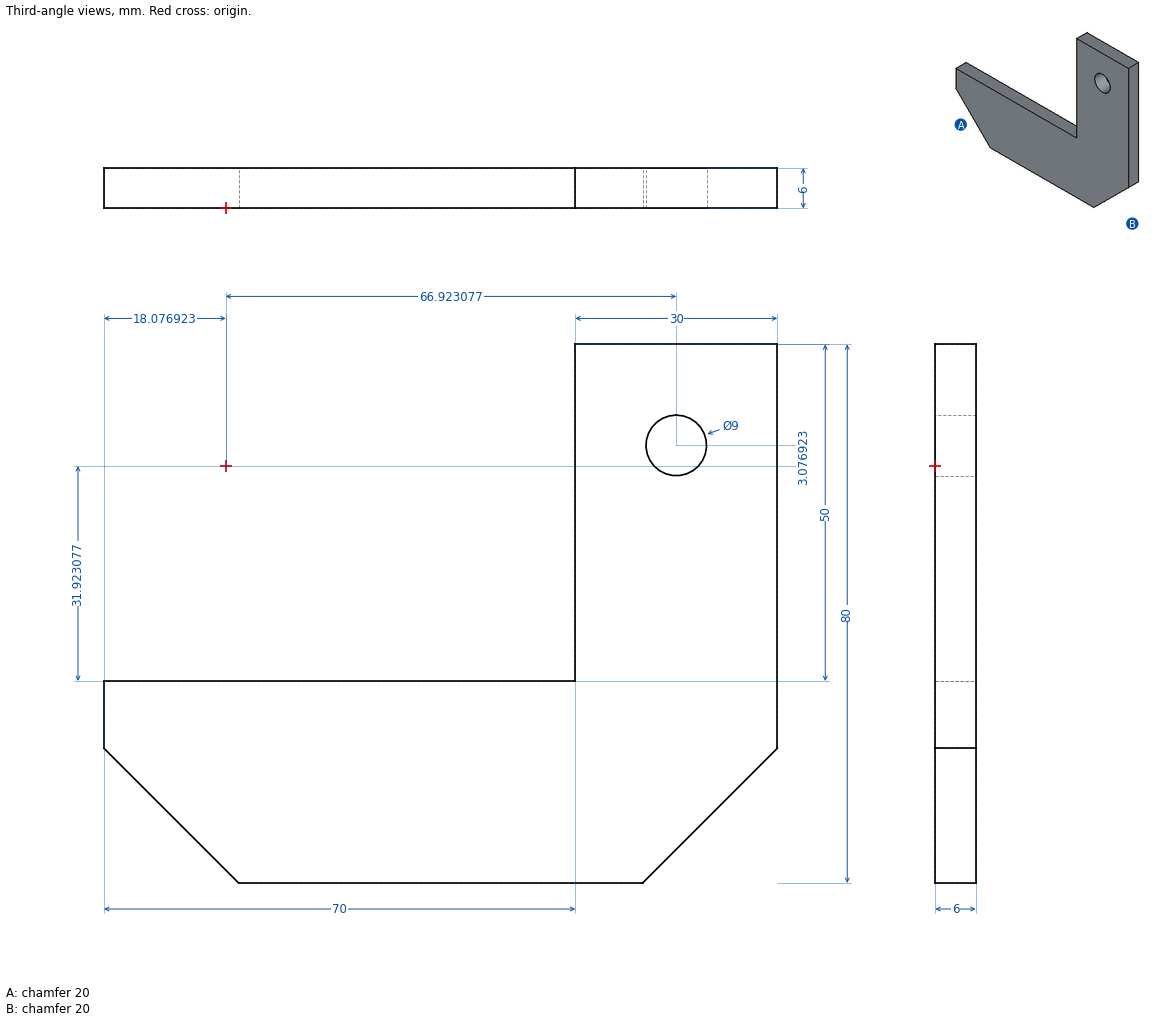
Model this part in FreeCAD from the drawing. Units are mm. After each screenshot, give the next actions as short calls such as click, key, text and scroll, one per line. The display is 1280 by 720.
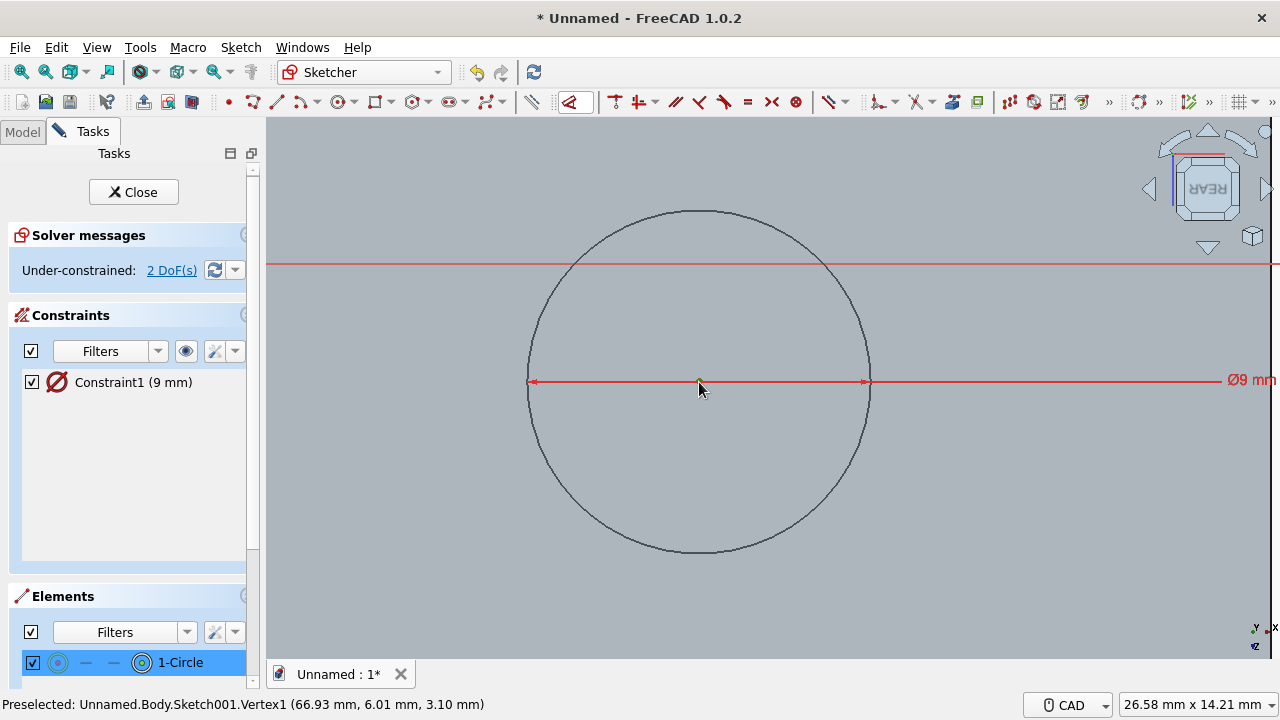
key(i)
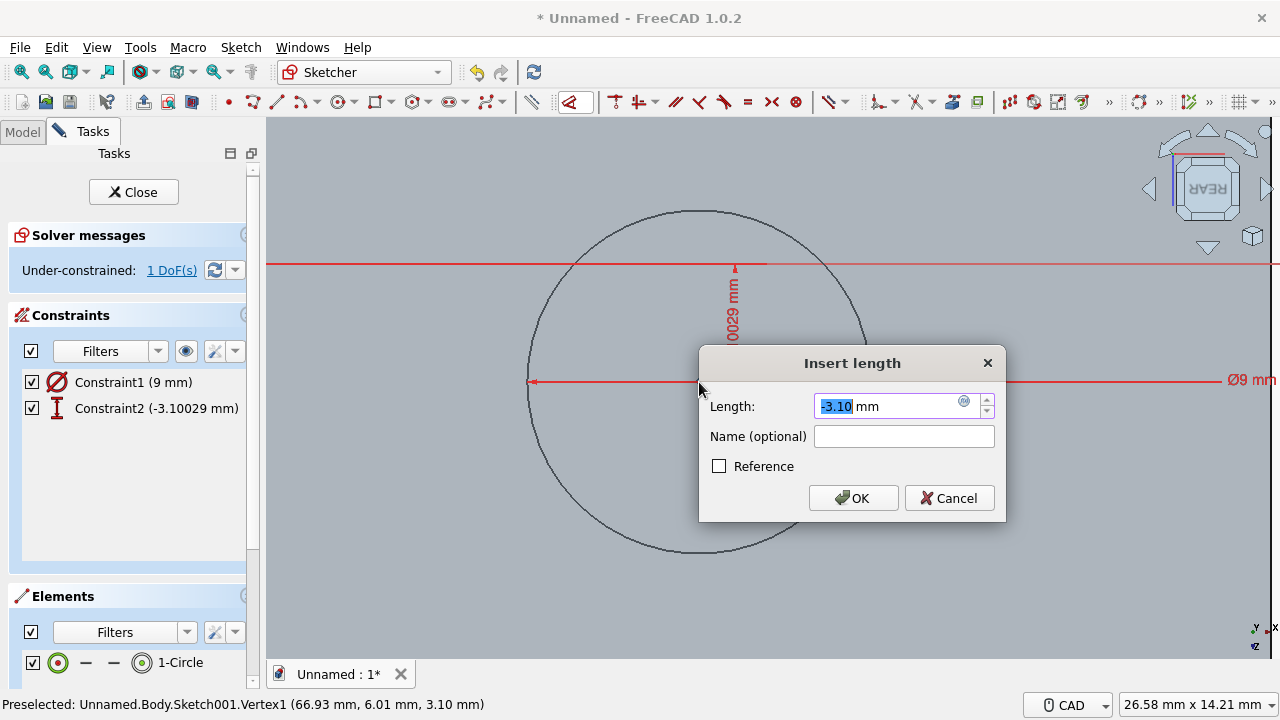
text(-3.076923)
key(Return)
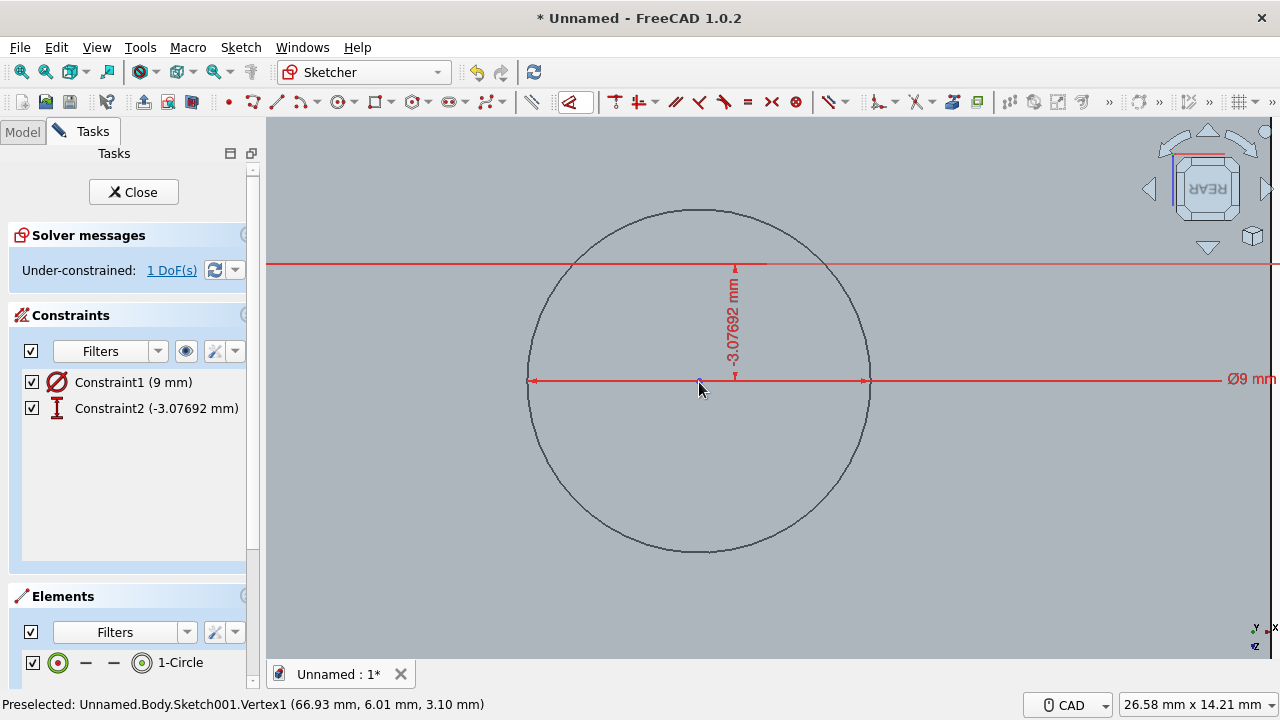
click(699, 381)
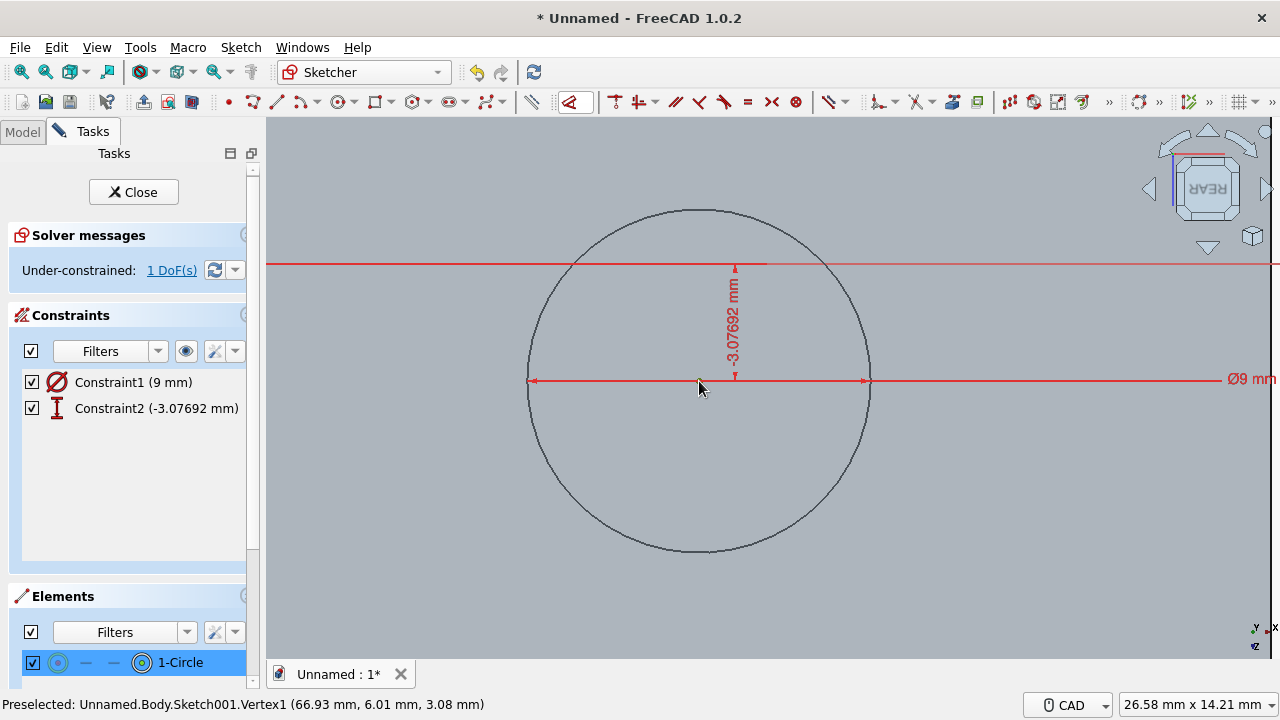
key(l)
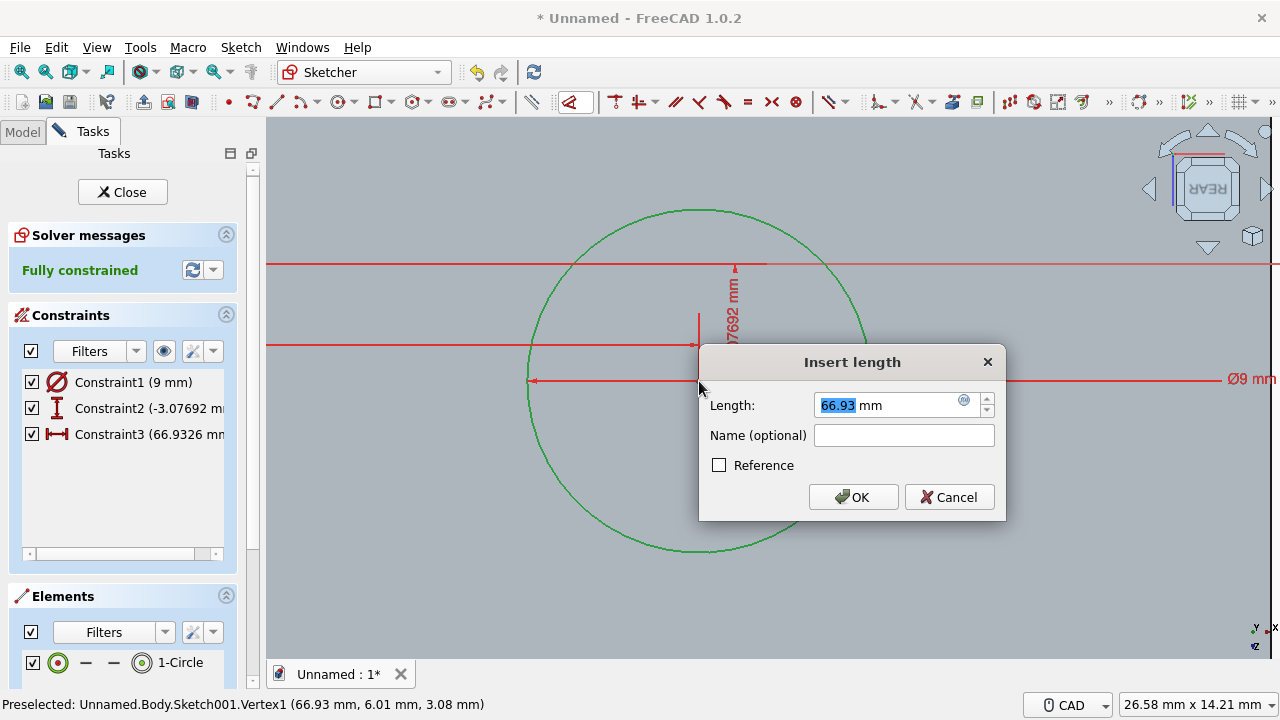
text(66.923077)
key(Return)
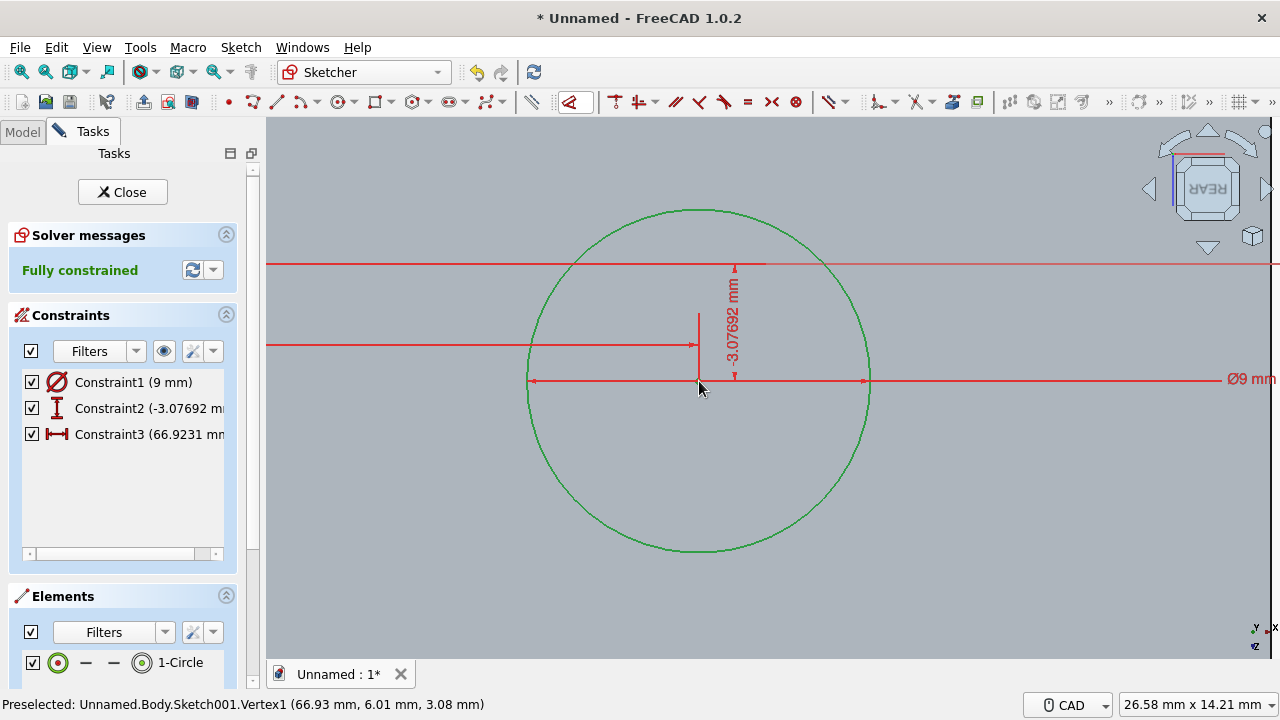
click(123, 192)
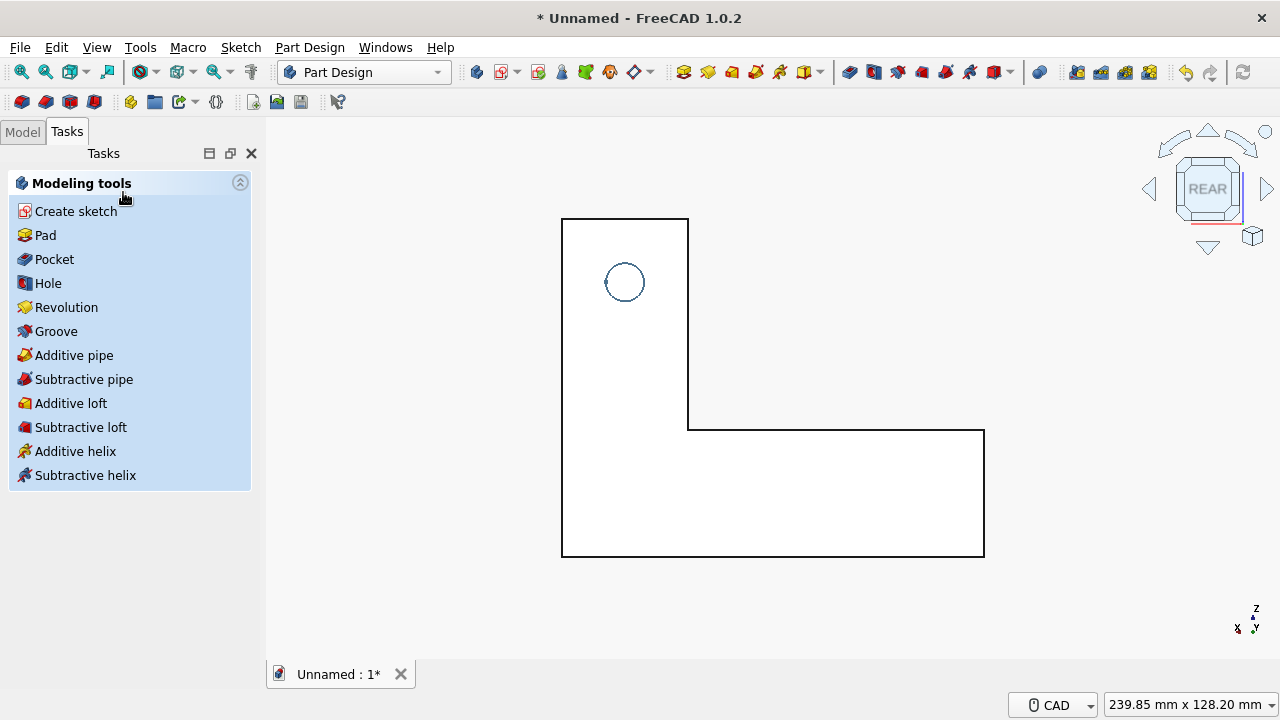
click(850, 72)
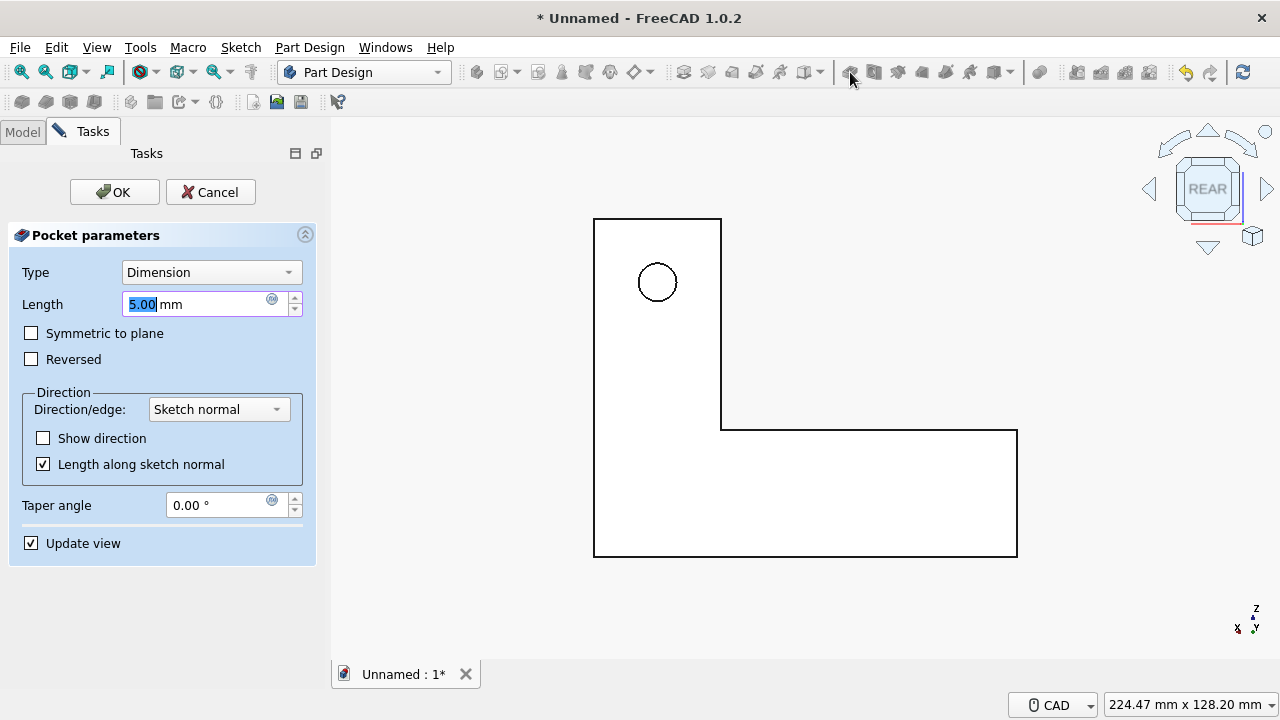
text(6)
key(Tab)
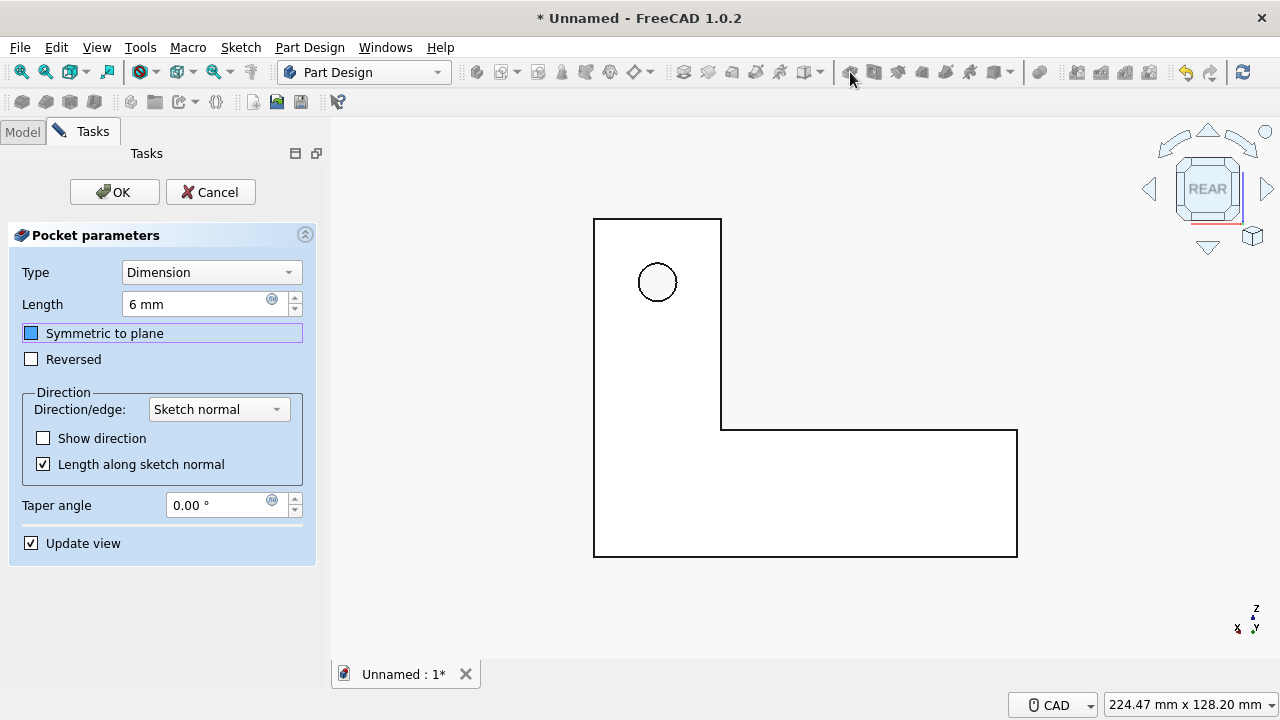
click(115, 192)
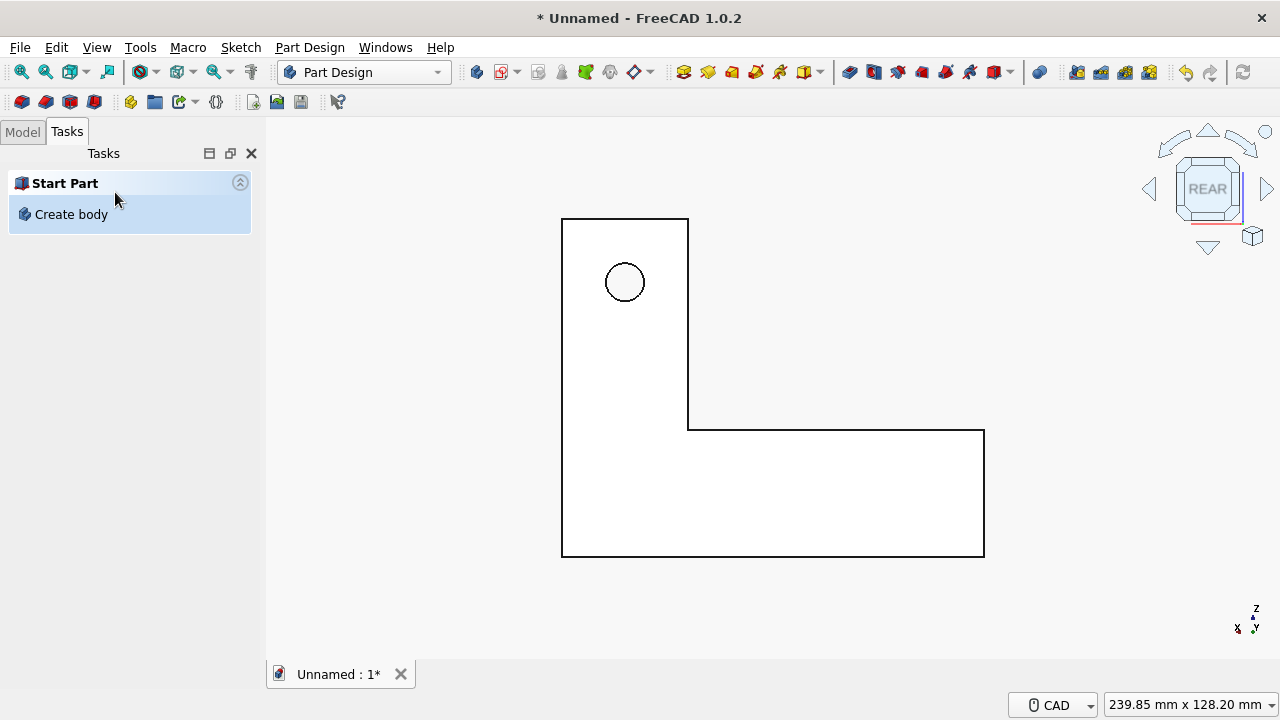
key(0)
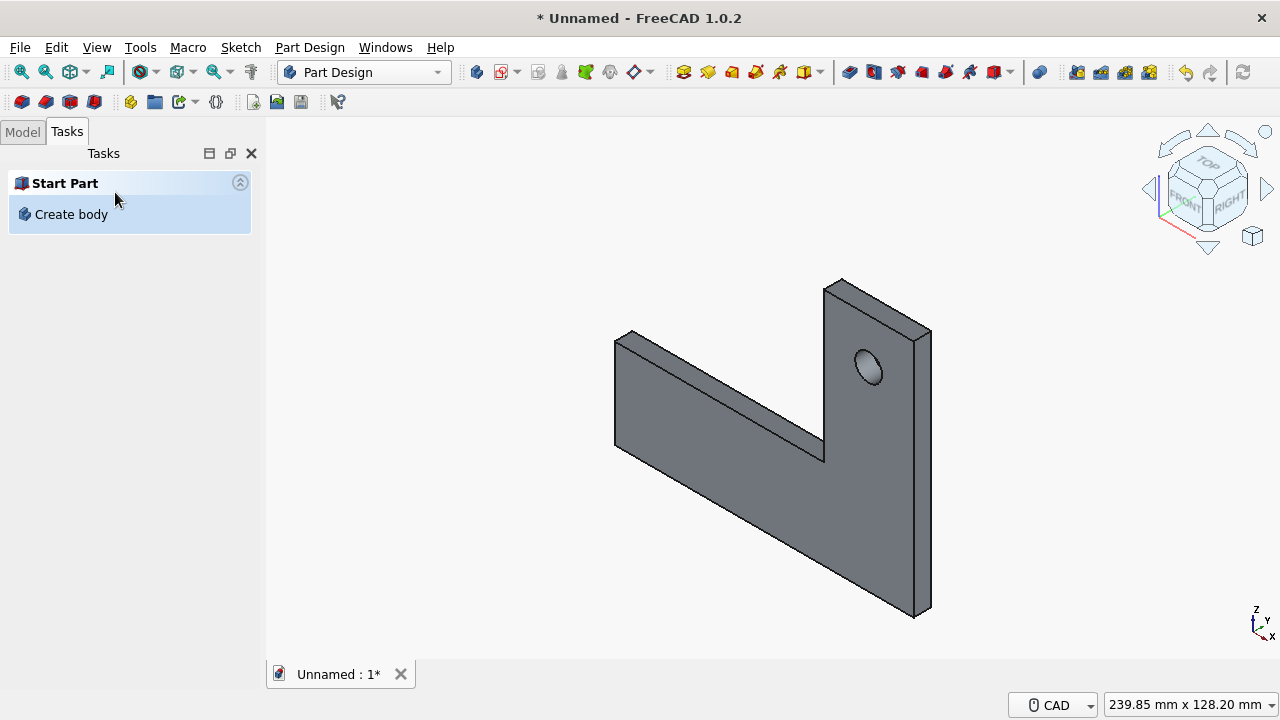
key(2)